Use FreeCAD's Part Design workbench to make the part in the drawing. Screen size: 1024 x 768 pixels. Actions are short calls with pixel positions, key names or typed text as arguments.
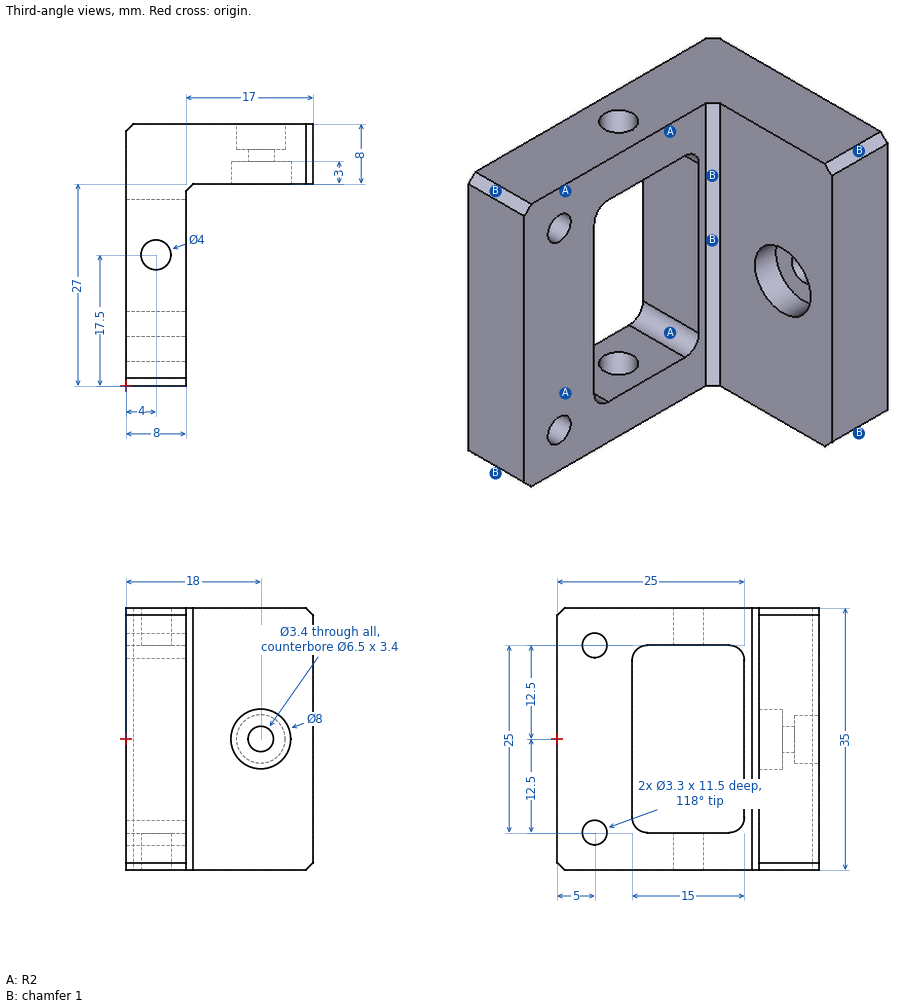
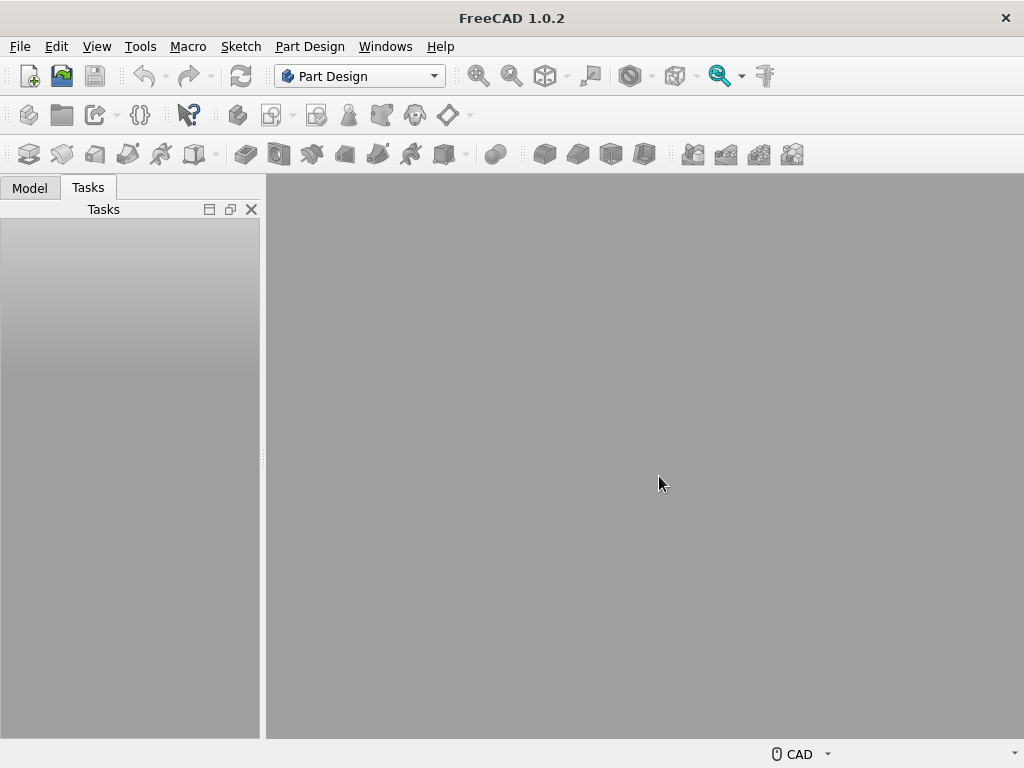
click(29, 76)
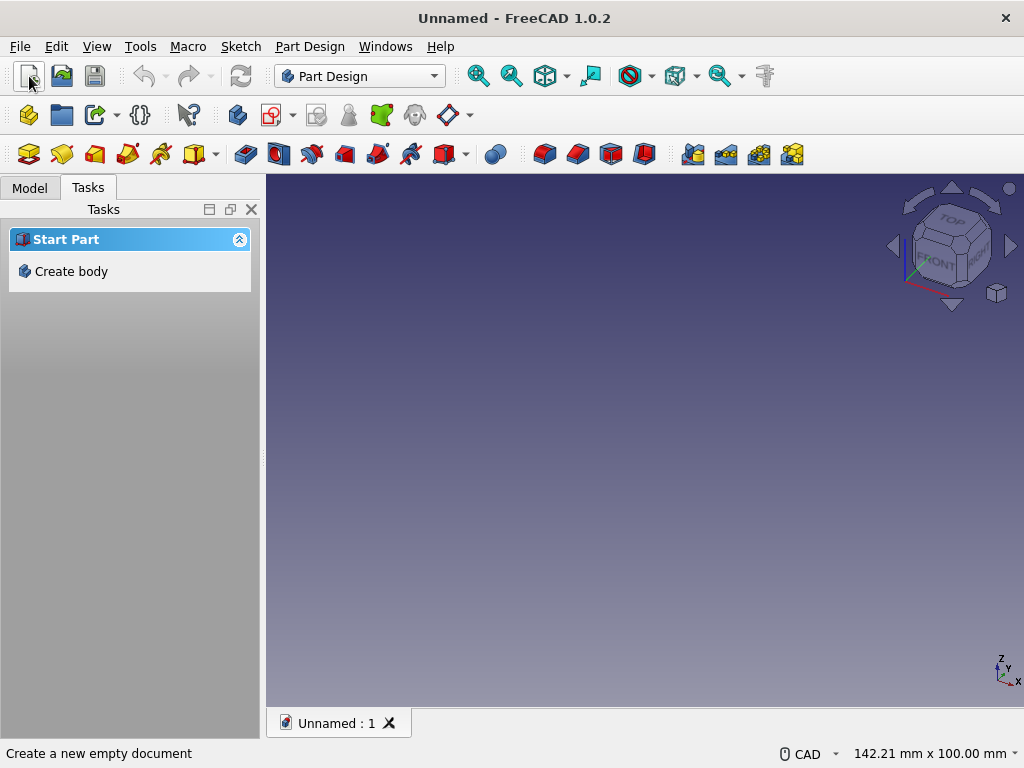
click(270, 116)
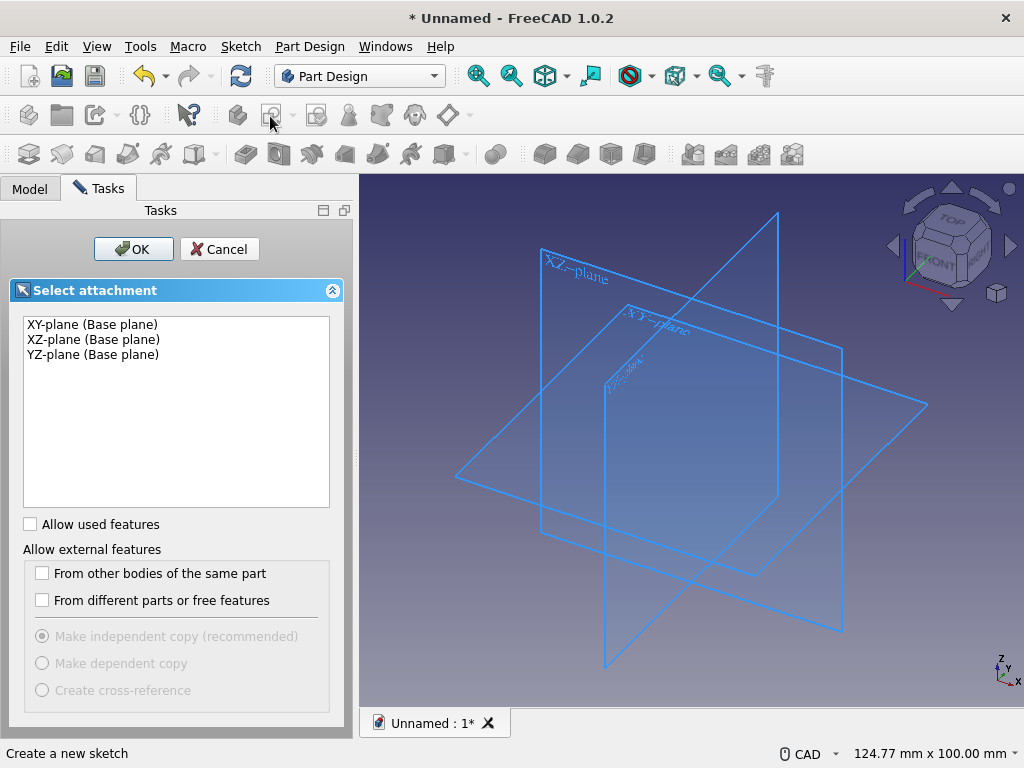
click(84, 324)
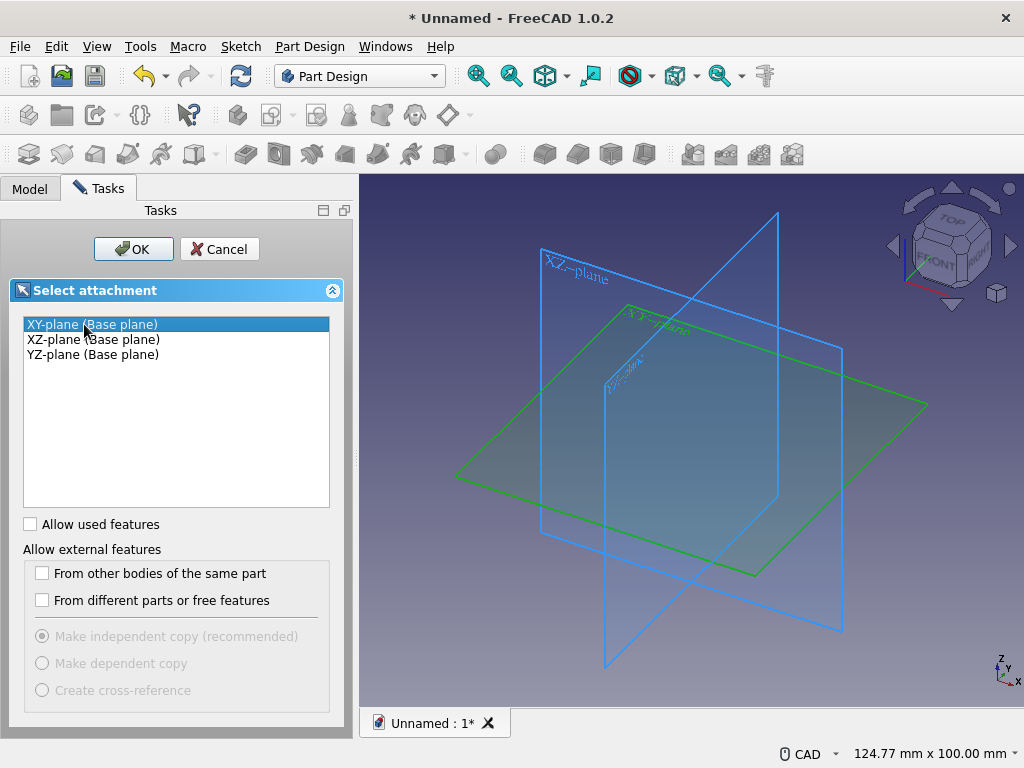
click(134, 249)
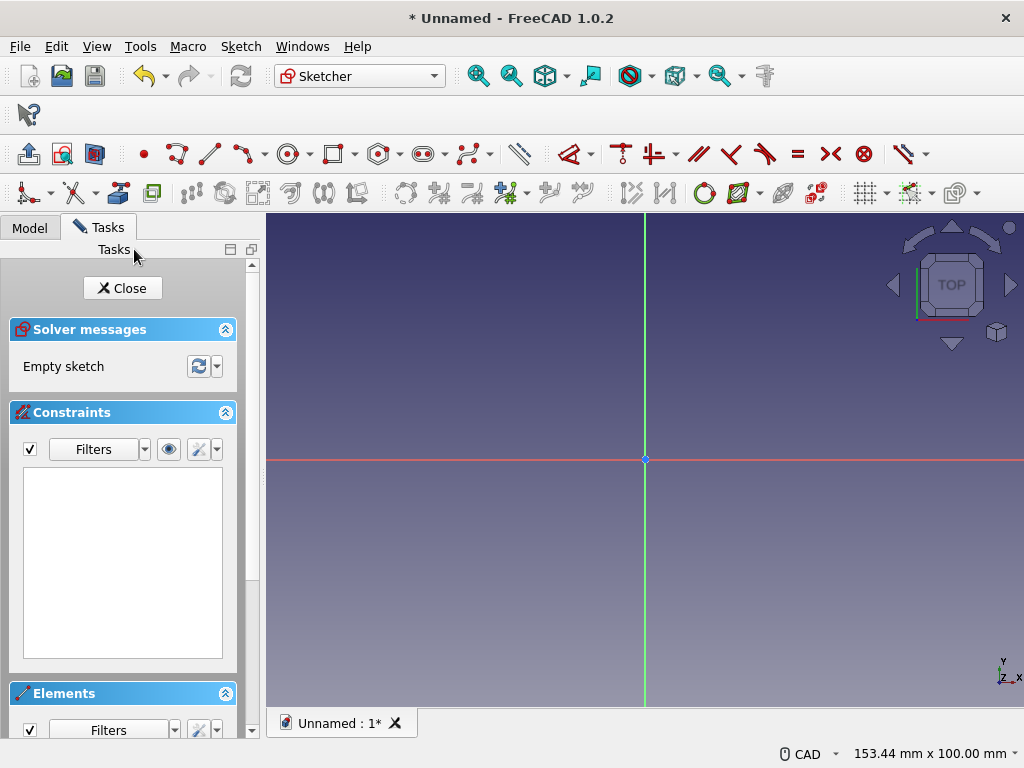
scroll(859, 268, up, 3)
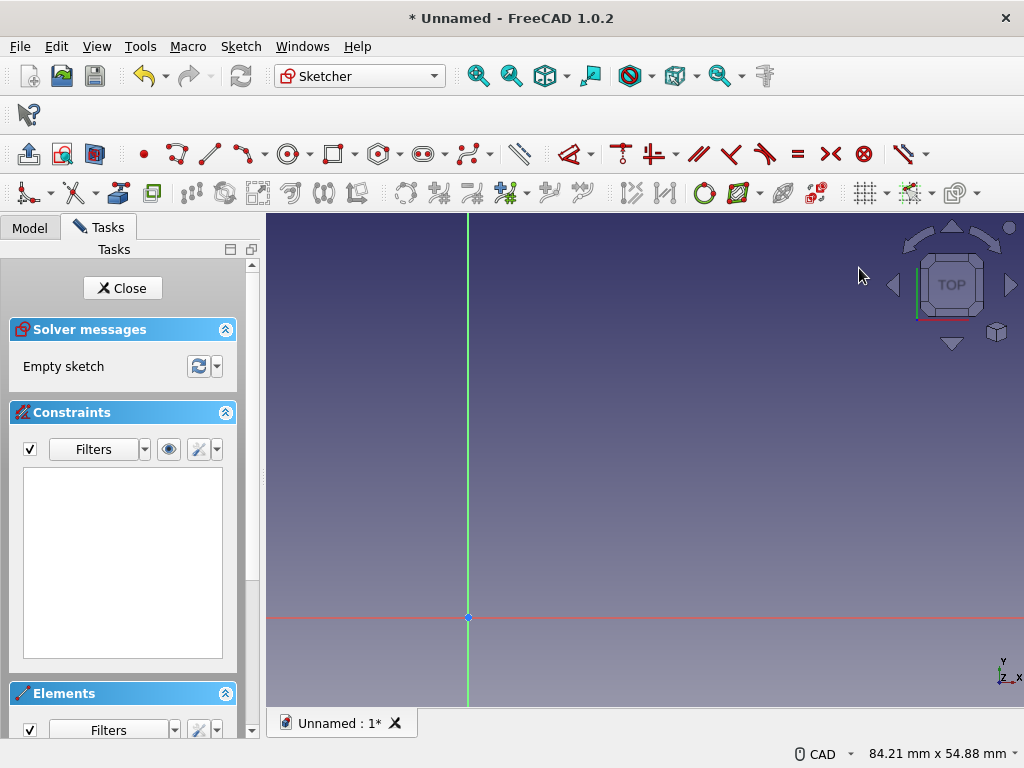
click(177, 154)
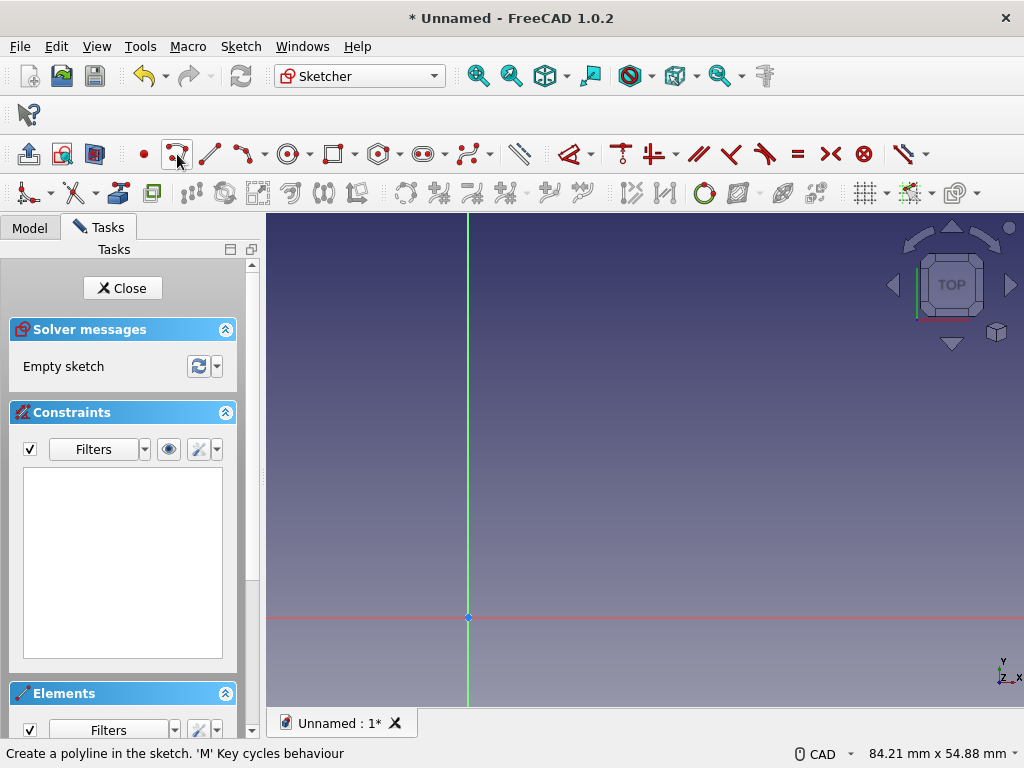
click(468, 618)
click(540, 609)
click(540, 375)
click(693, 375)
click(693, 303)
click(477, 303)
click(468, 618)
key(Escape)
key(Escape)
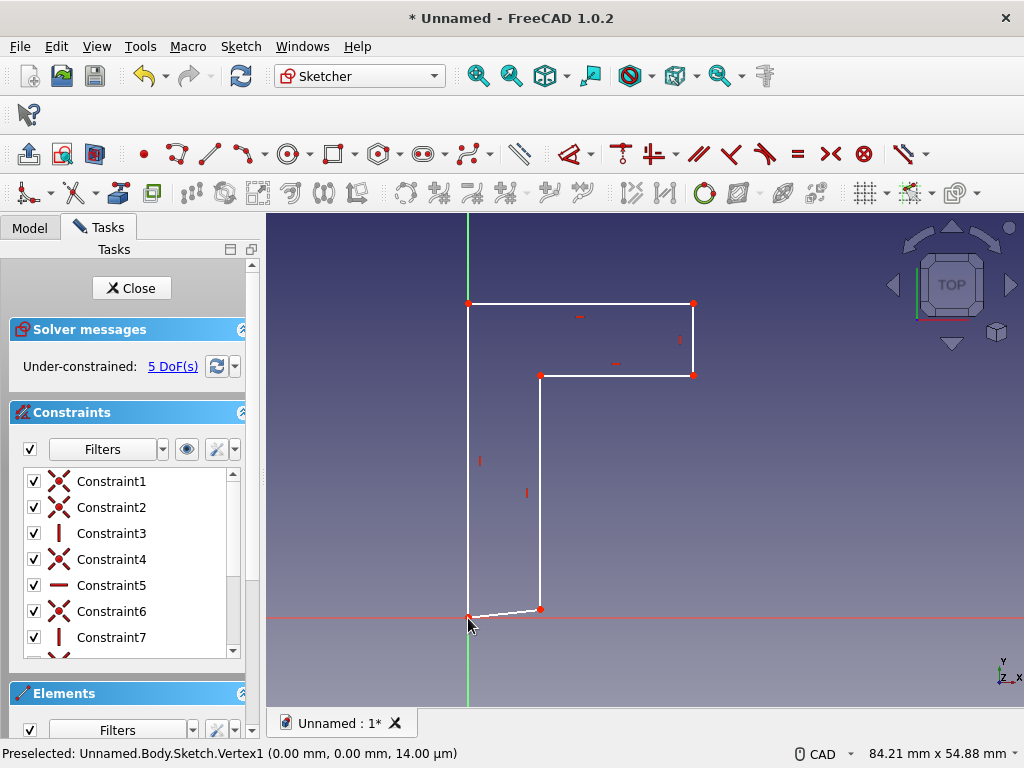
click(490, 615)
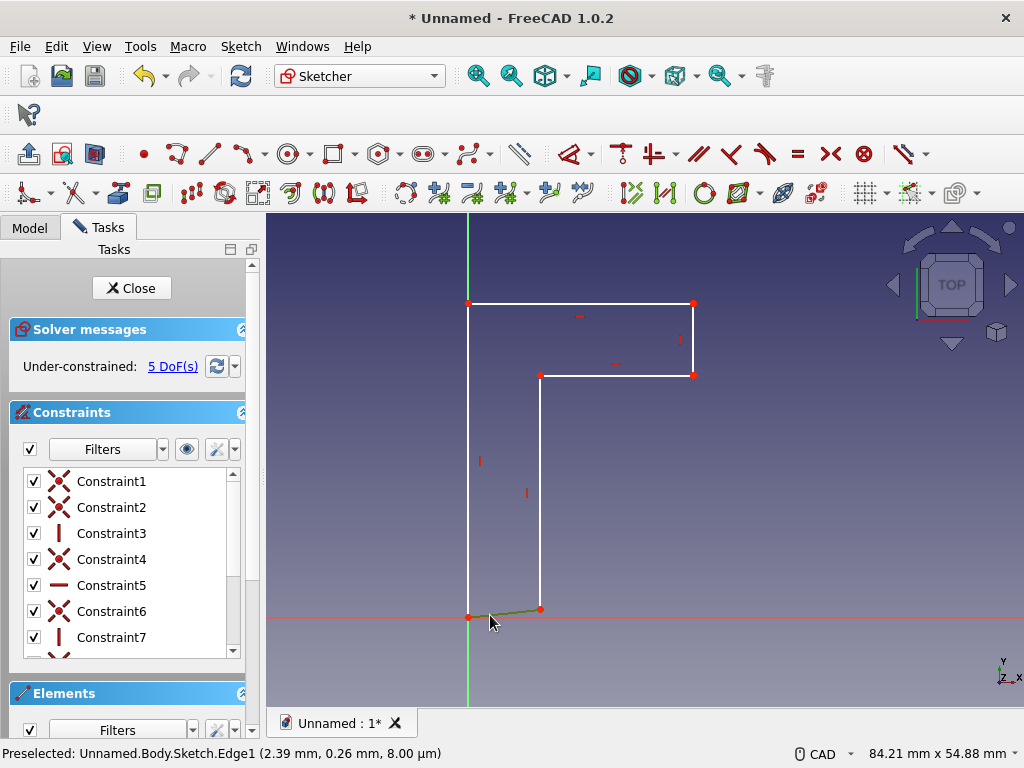
key(h)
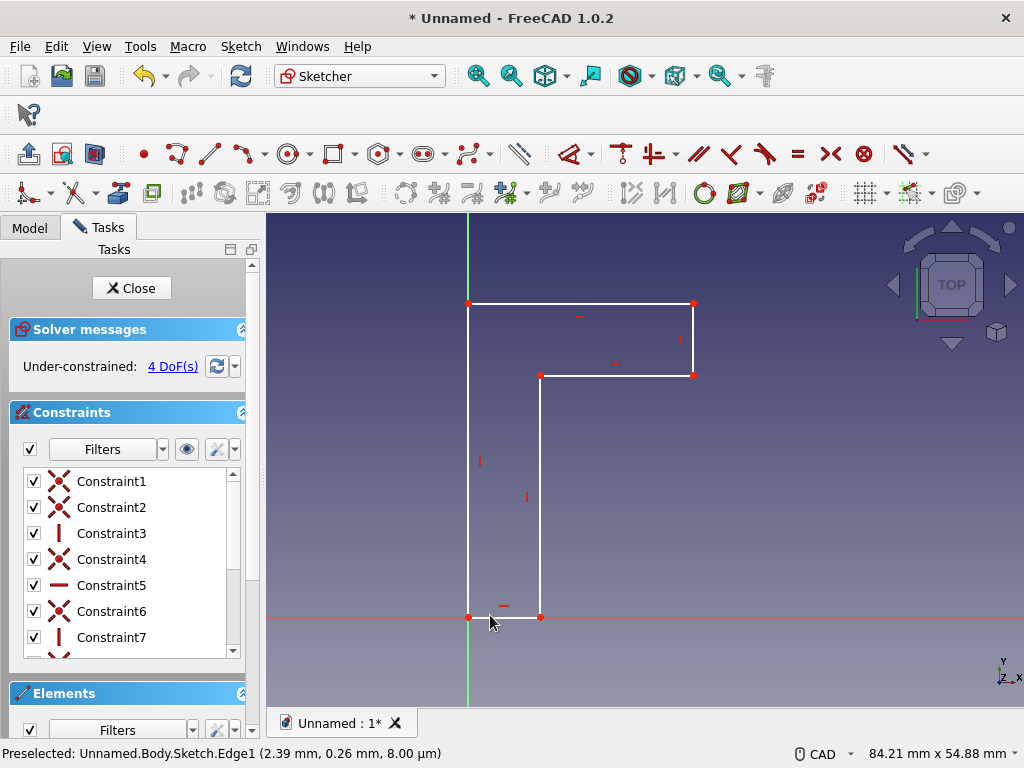
key(d)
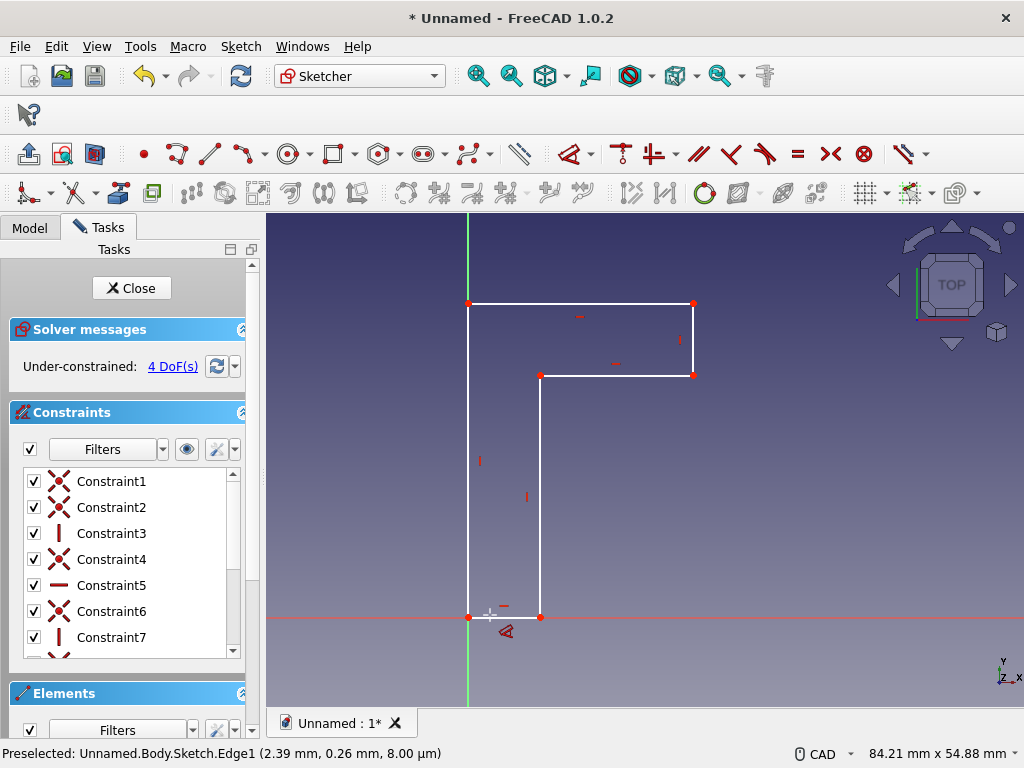
click(490, 618)
click(504, 652)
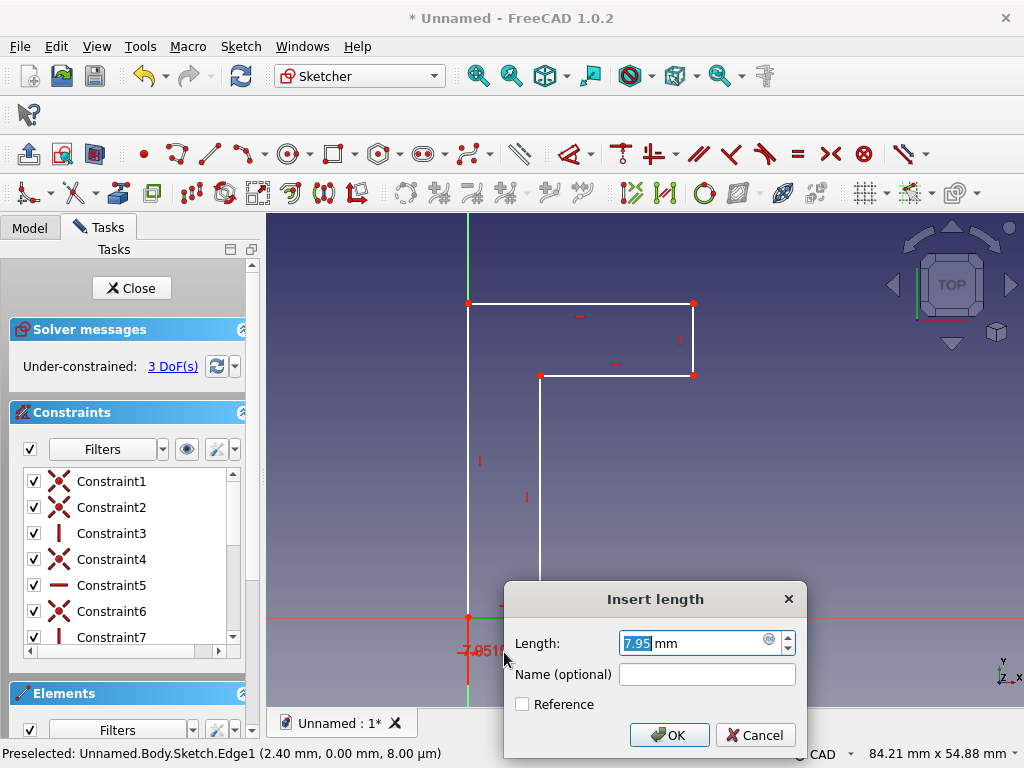
text(8)
key(Return)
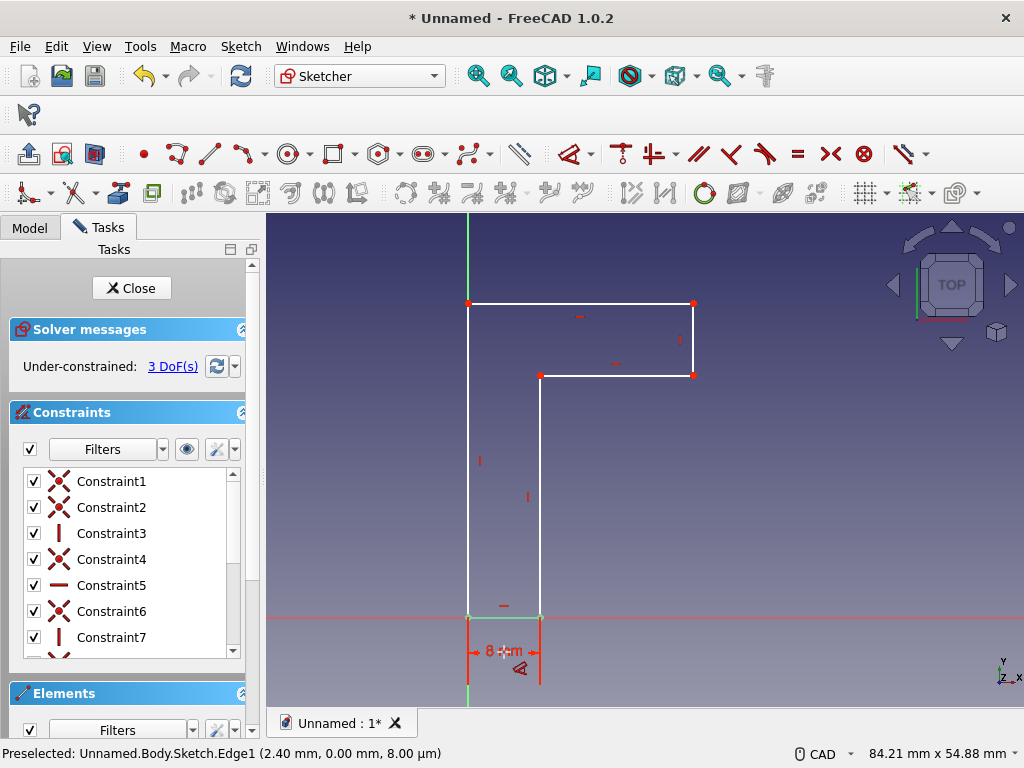
click(693, 354)
click(727, 340)